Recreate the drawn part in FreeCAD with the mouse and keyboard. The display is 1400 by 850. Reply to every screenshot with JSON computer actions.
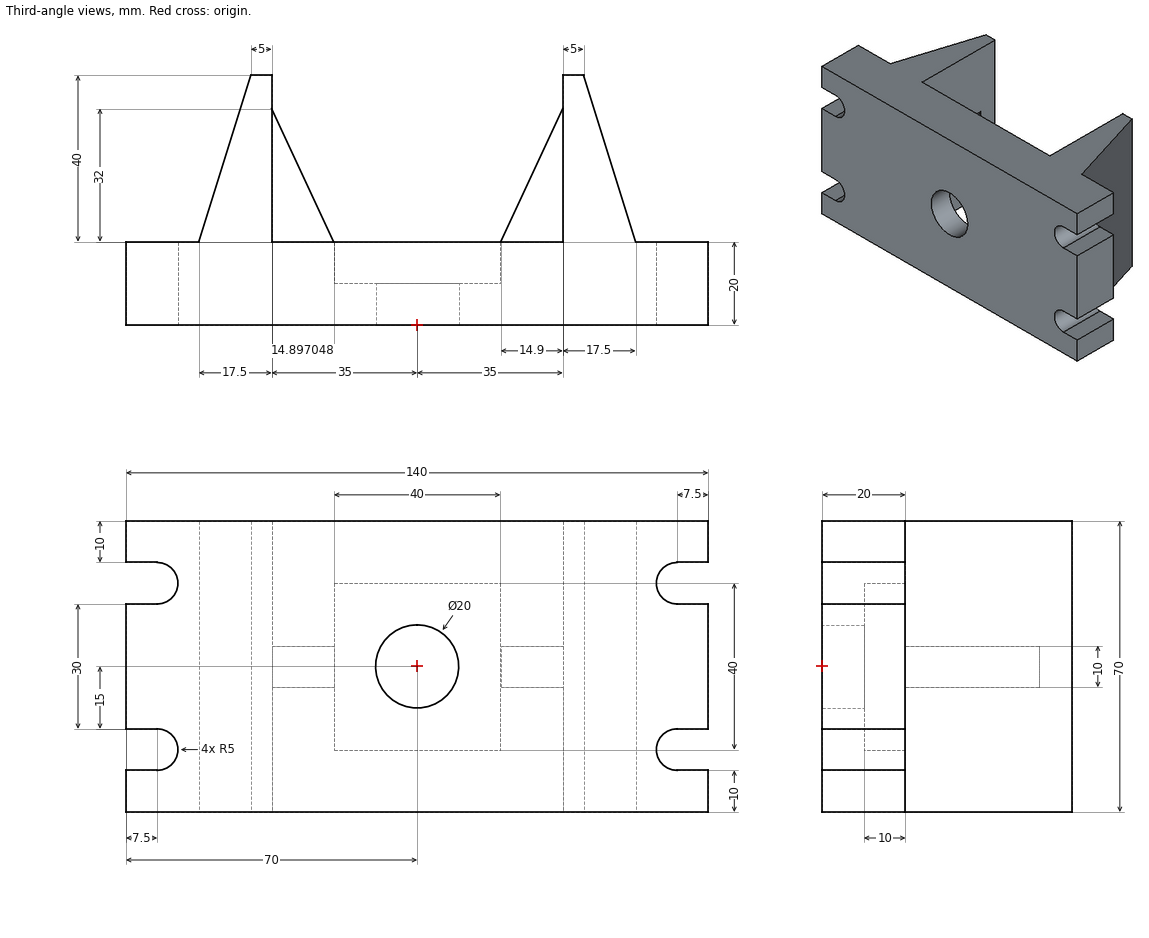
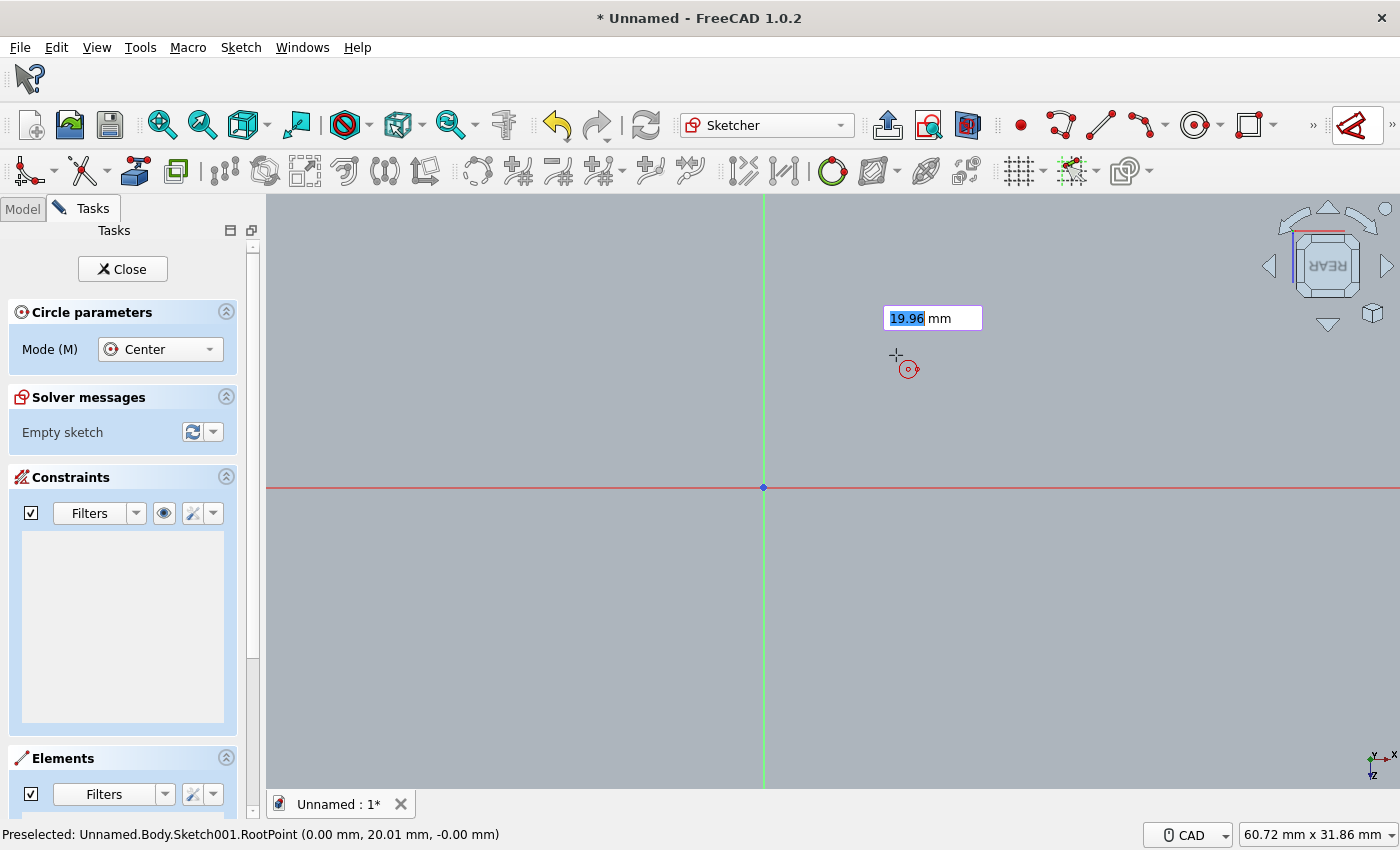
{"action": "type", "text": "20"}
{"action": "key", "text": "Return"}
{"action": "key", "text": "Escape"}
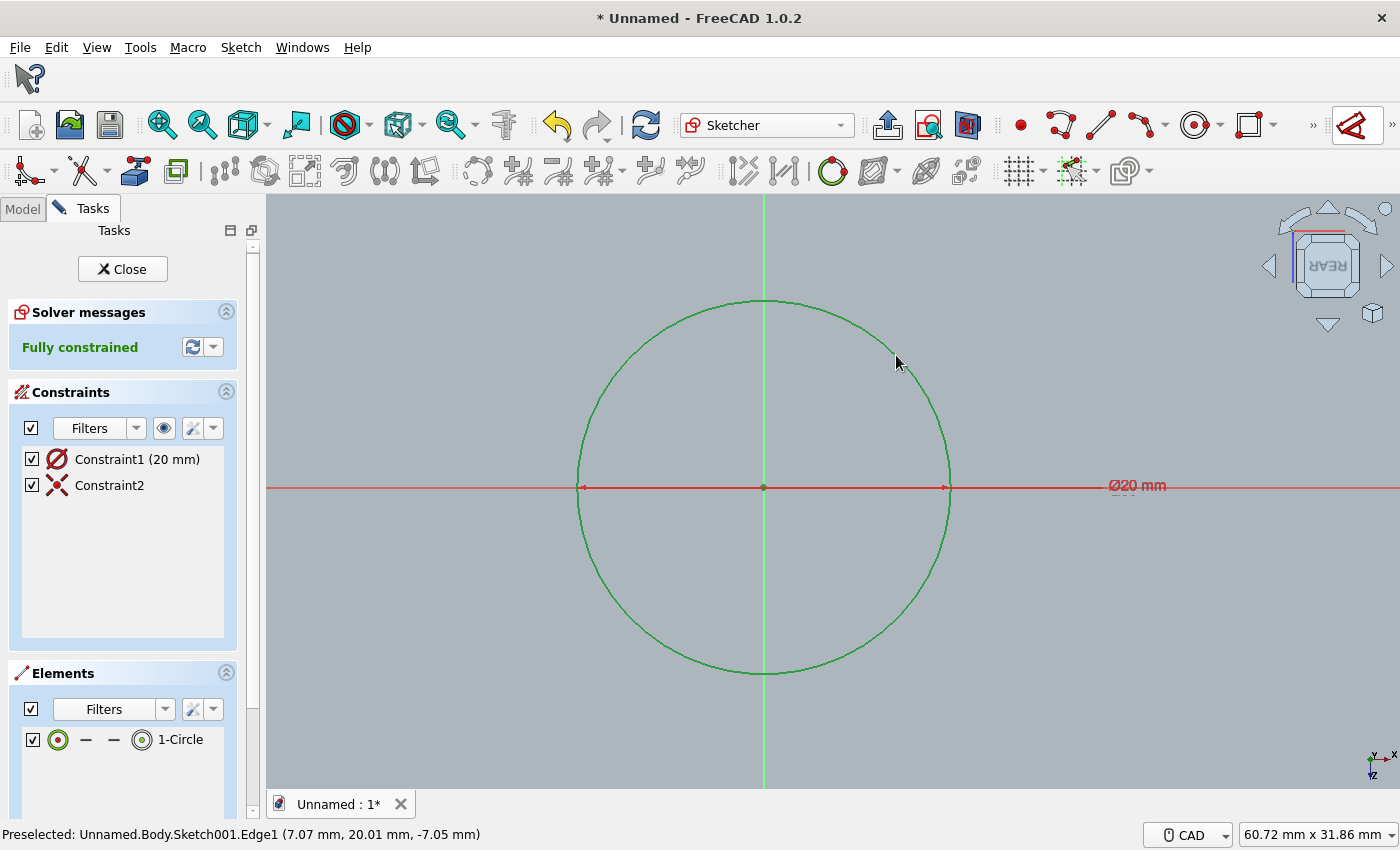
{"action": "left_click", "coordinate": [123, 269]}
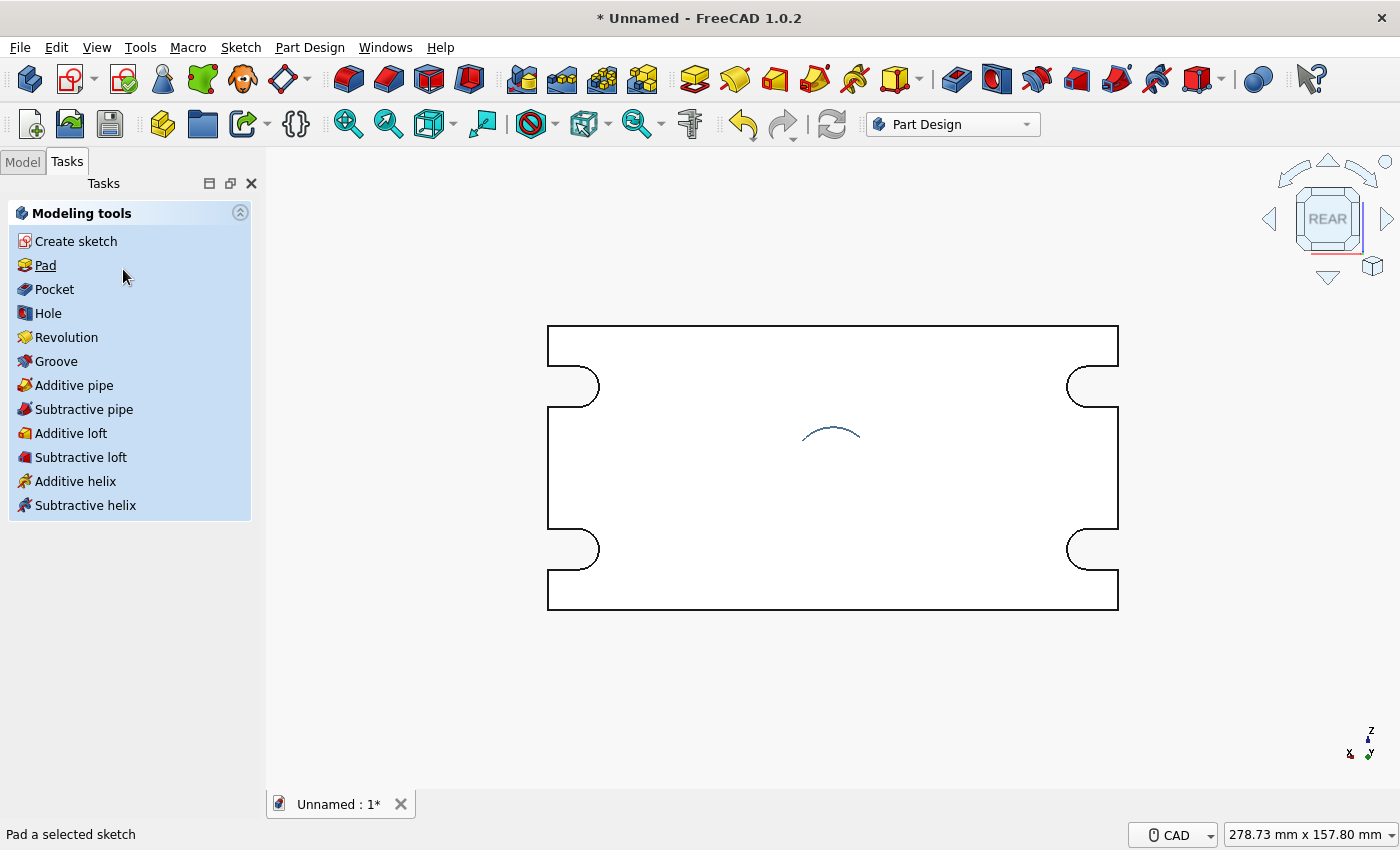
{"action": "left_click", "coordinate": [958, 80]}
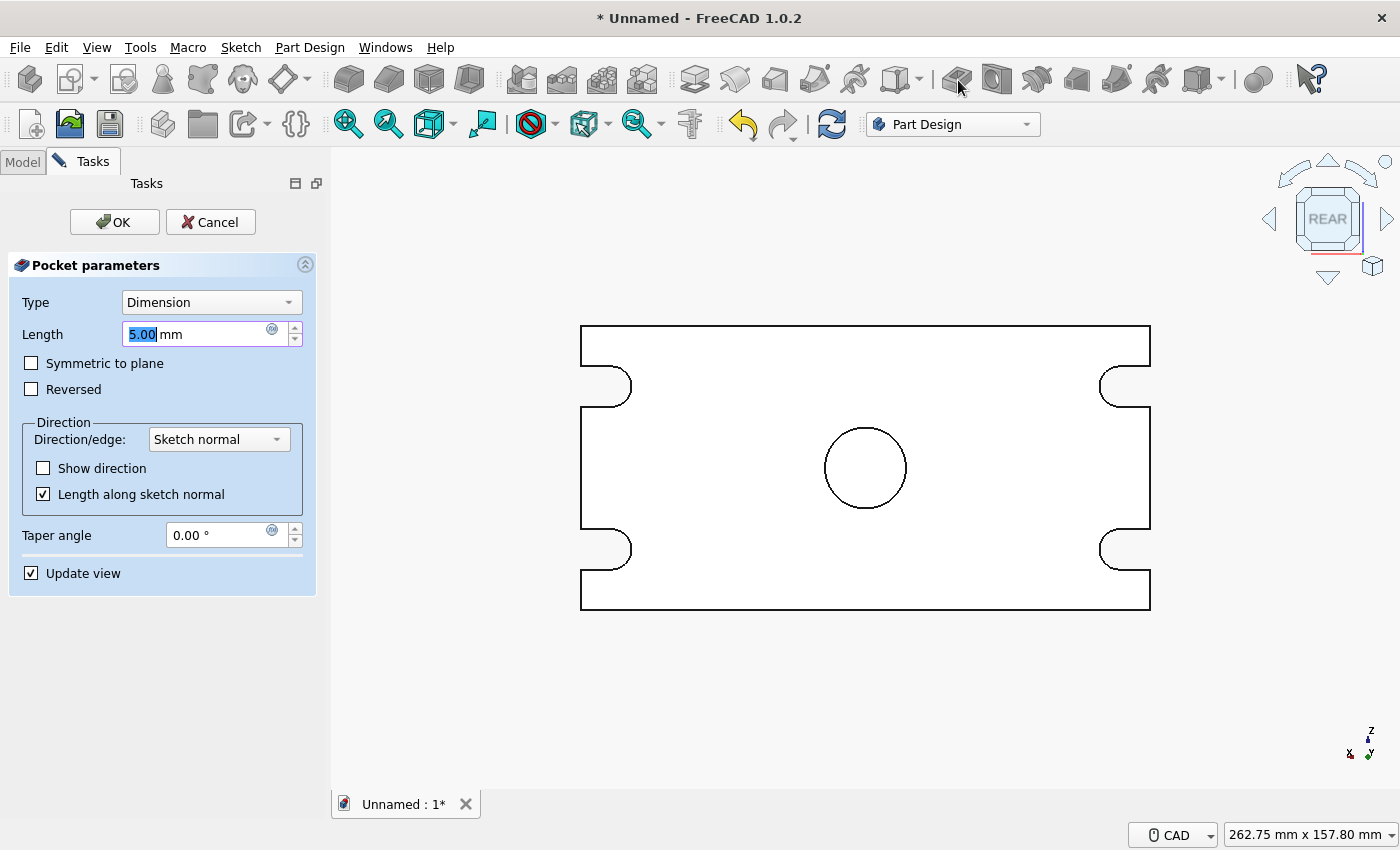
{"action": "type", "text": "20"}
{"action": "key", "text": "Tab"}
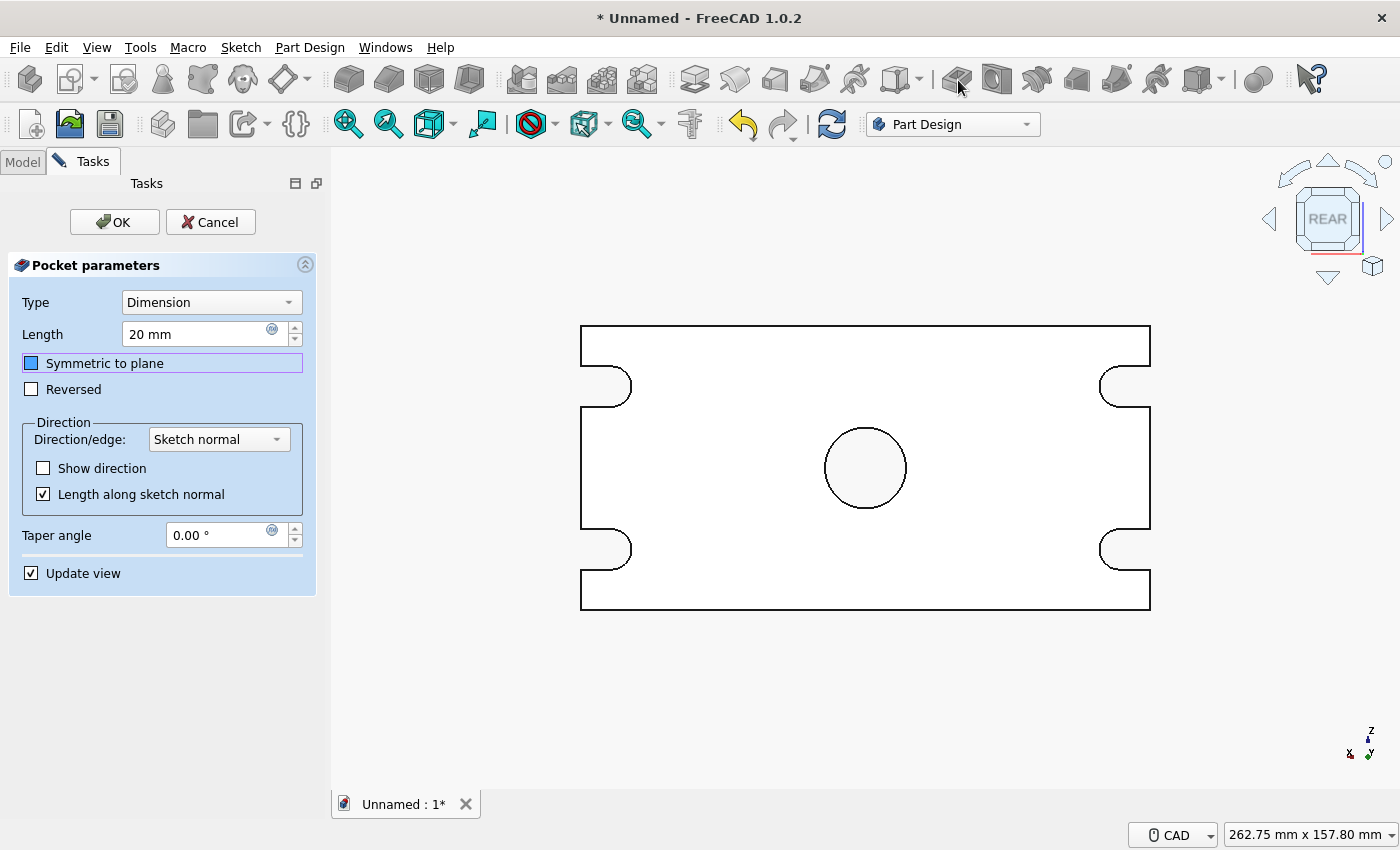
{"action": "left_click", "coordinate": [115, 222]}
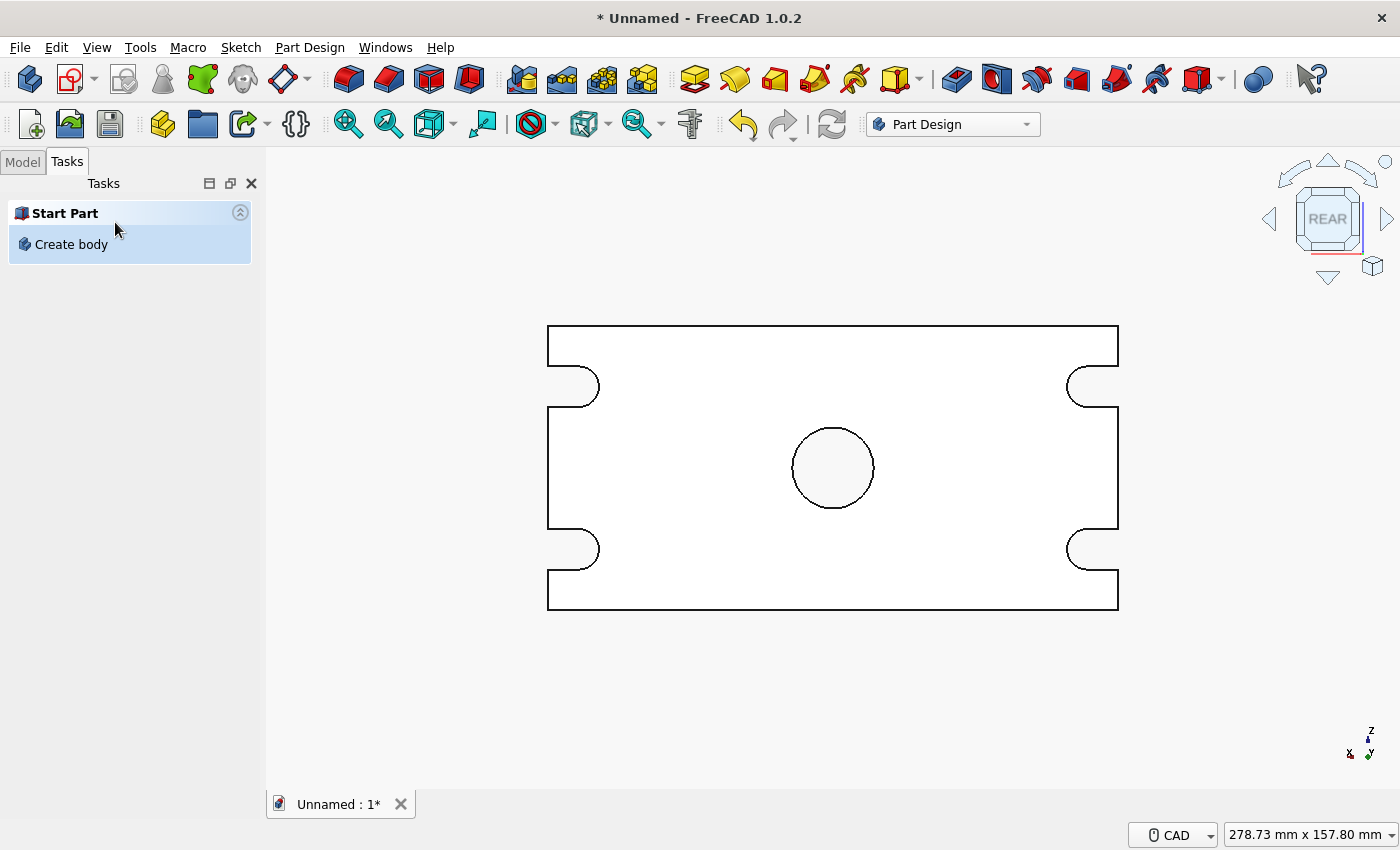
{"action": "left_click", "coordinate": [670, 467]}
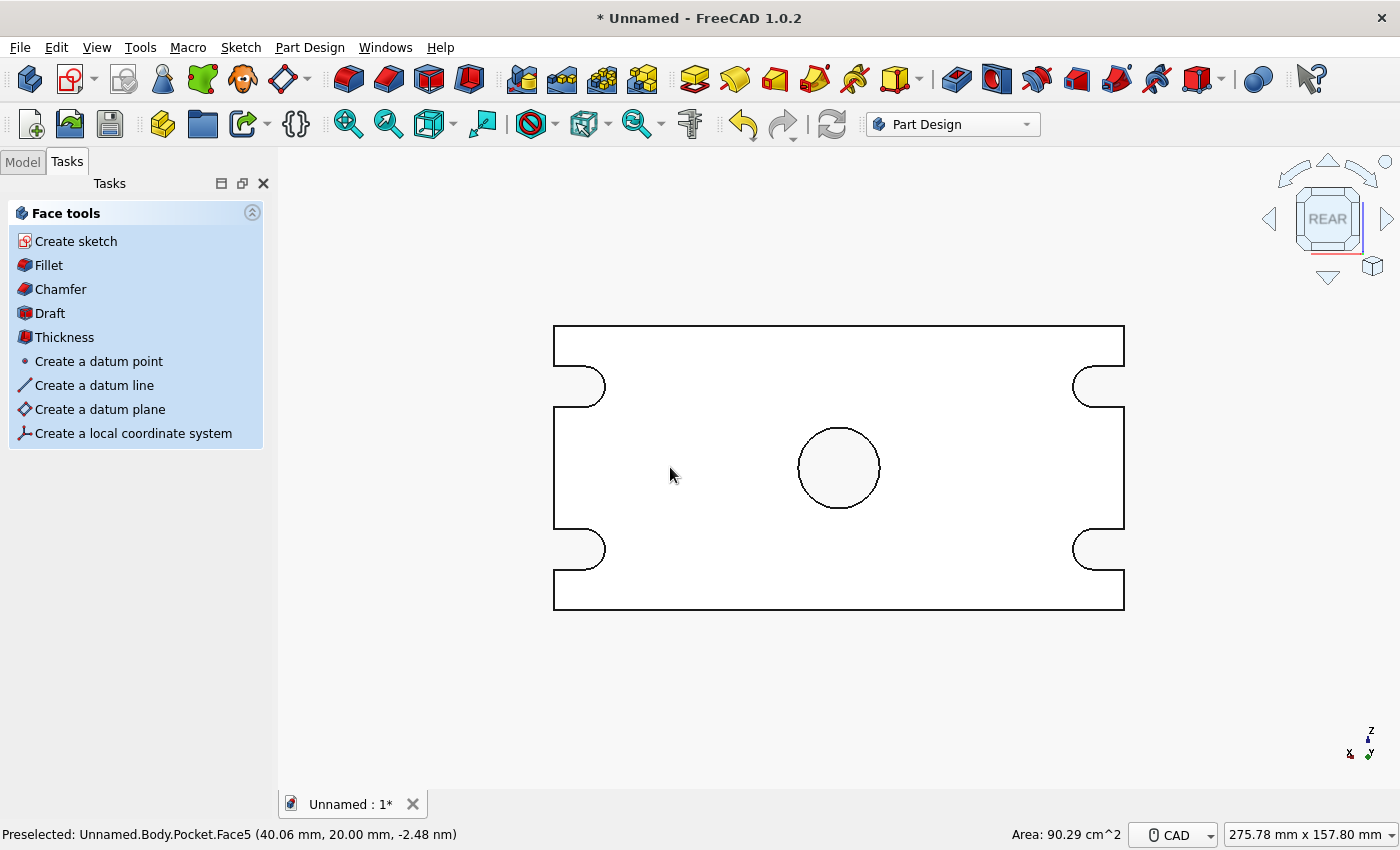
{"action": "left_click", "coordinate": [70, 80]}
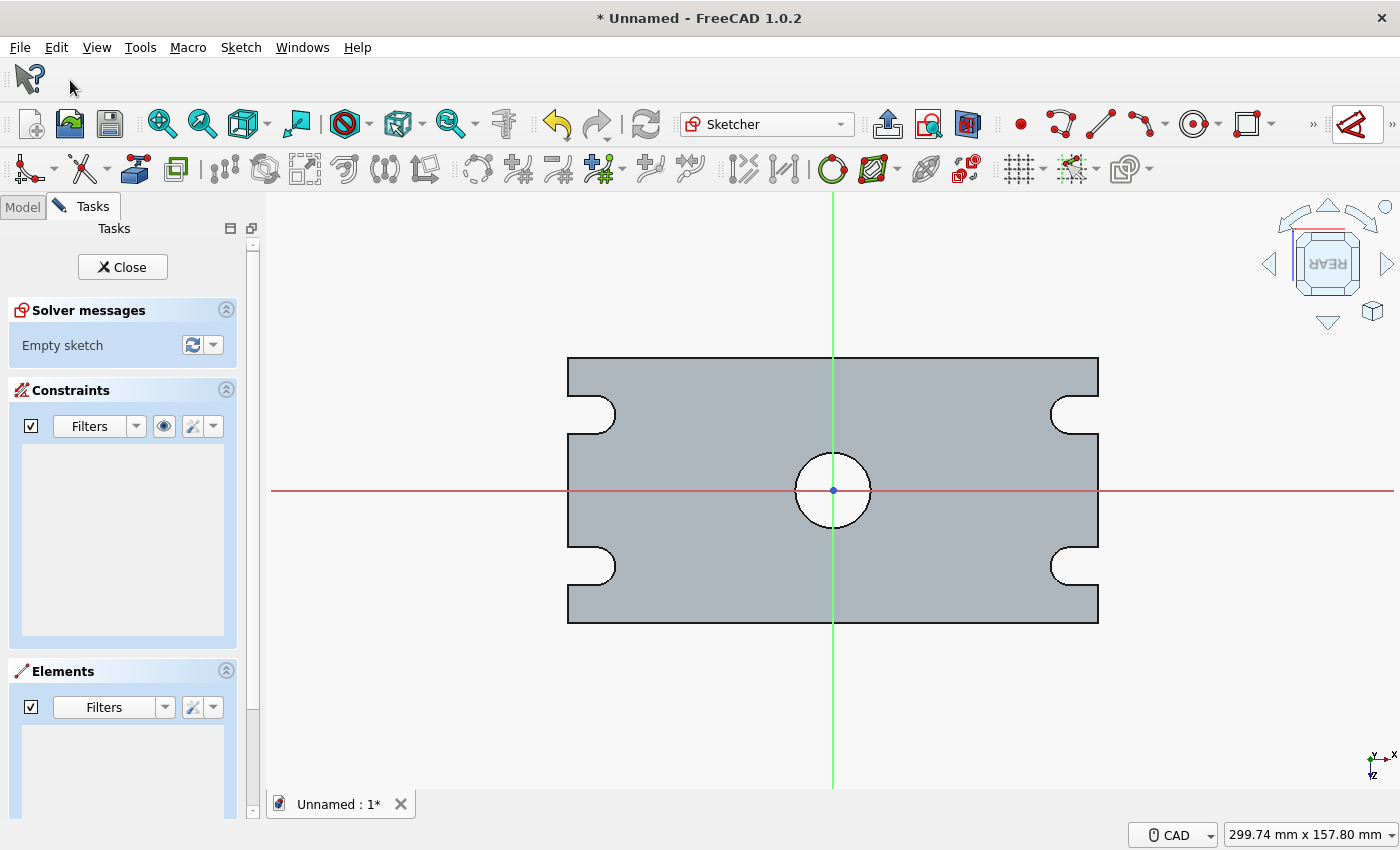
{"action": "scroll", "coordinate": [873, 490], "scroll_direction": "up", "scroll_amount": 5}